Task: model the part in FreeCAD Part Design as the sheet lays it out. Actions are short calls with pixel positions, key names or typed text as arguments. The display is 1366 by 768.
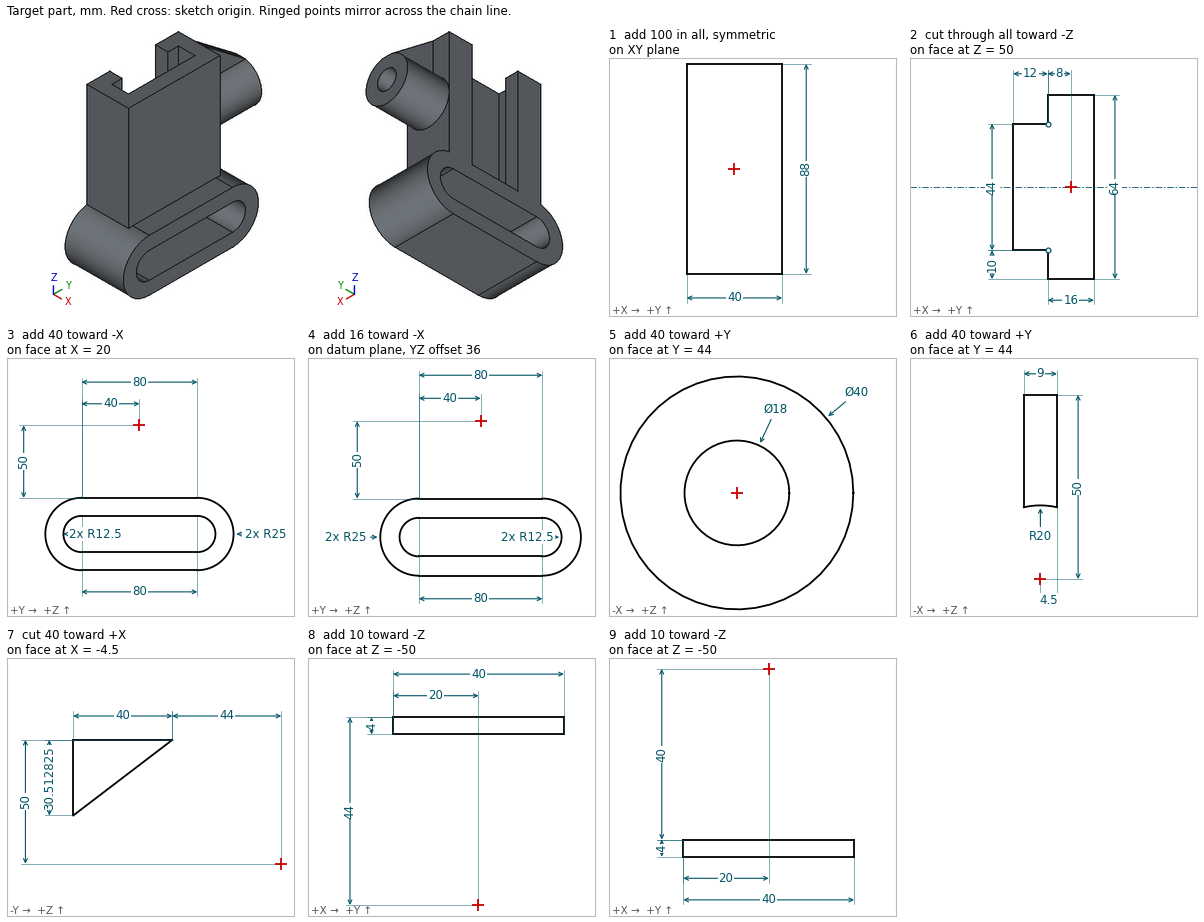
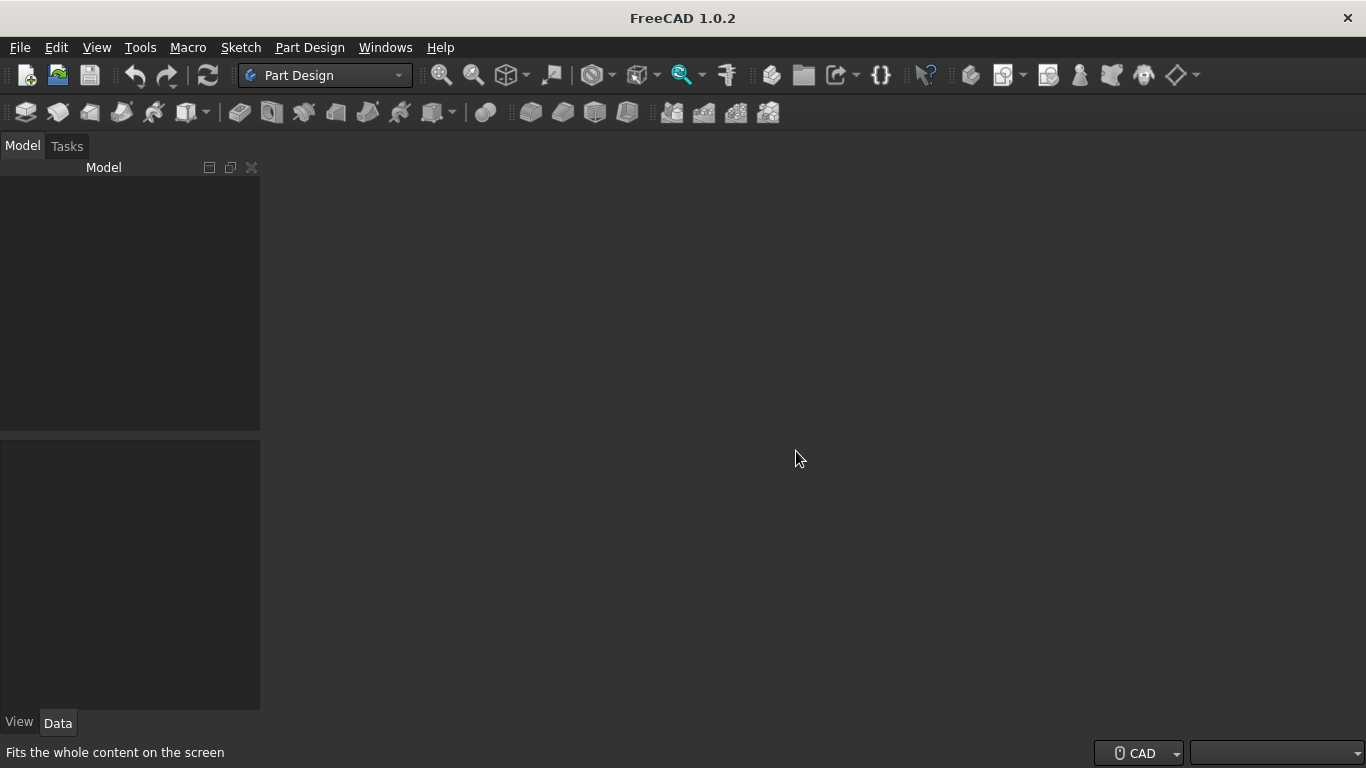
key(ctrl+n)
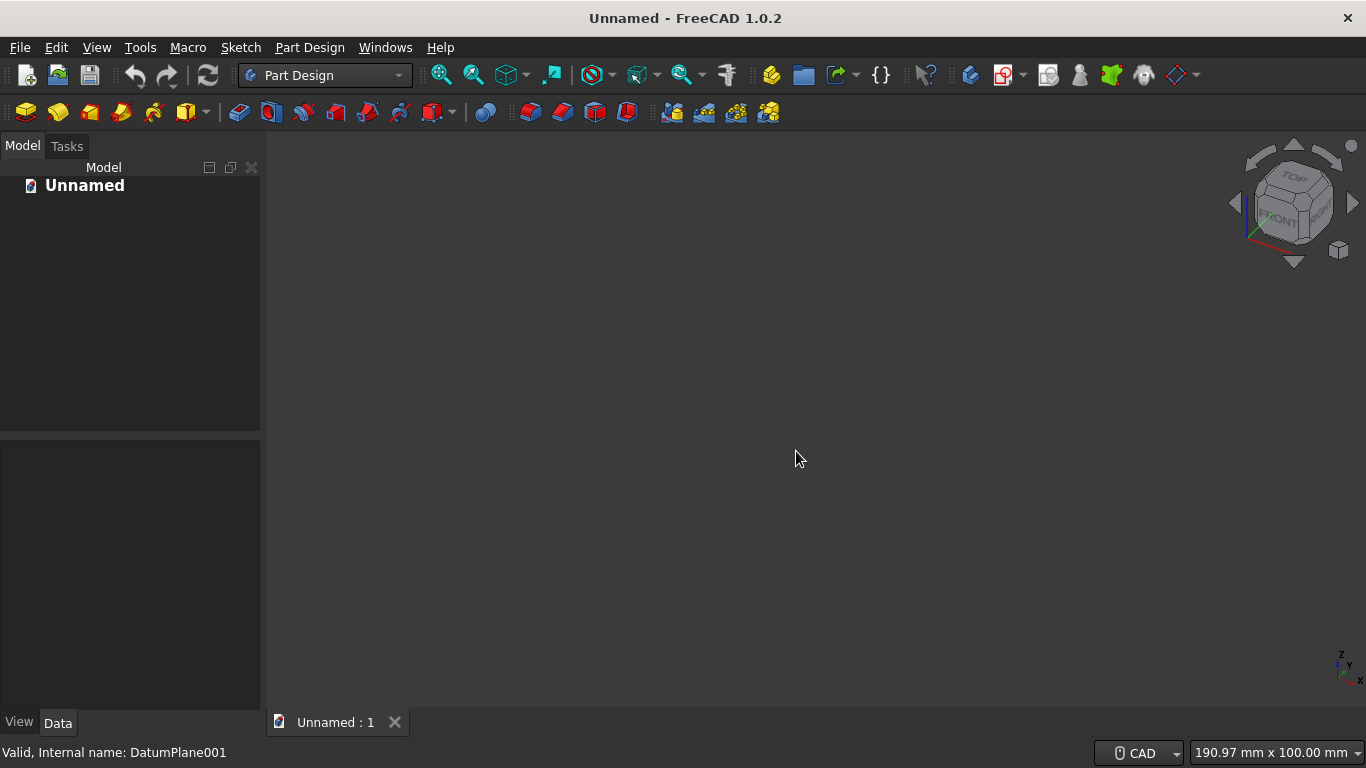
click(1004, 76)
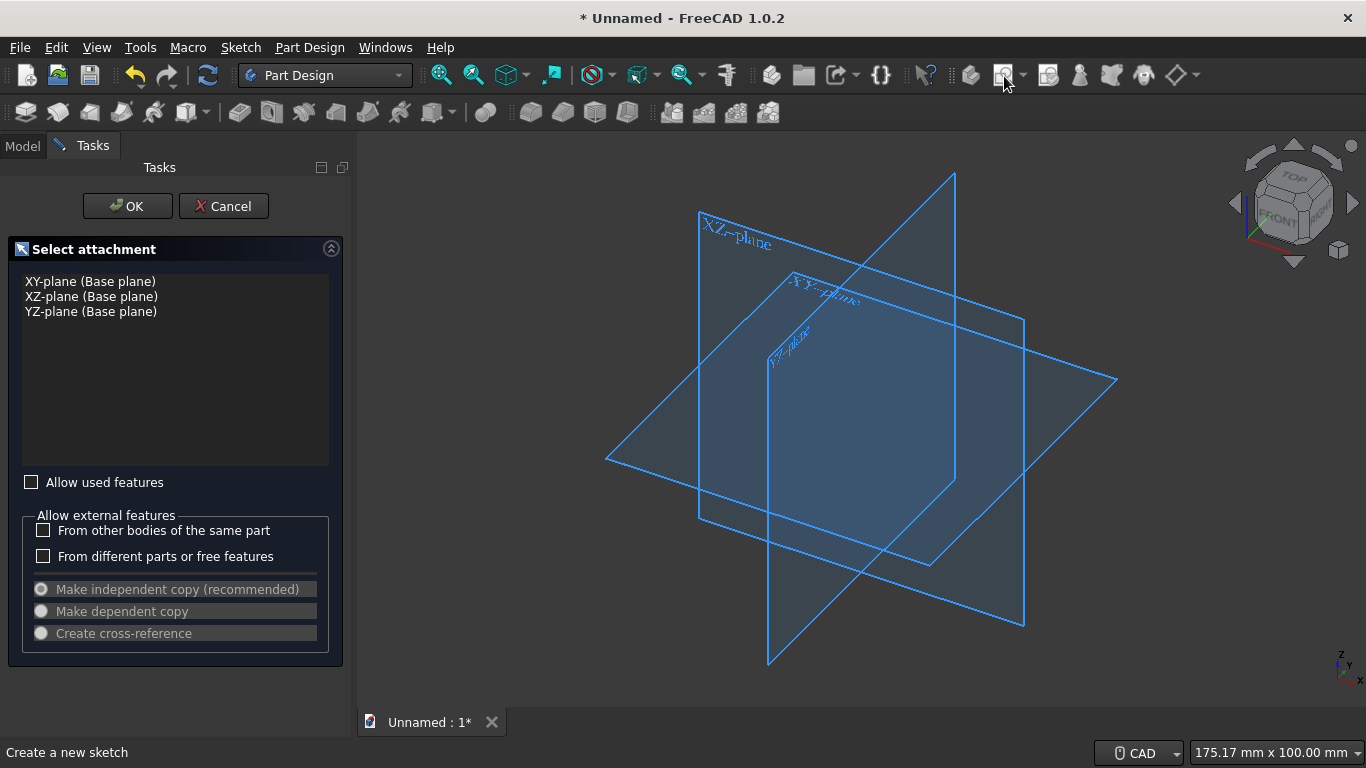
click(82, 282)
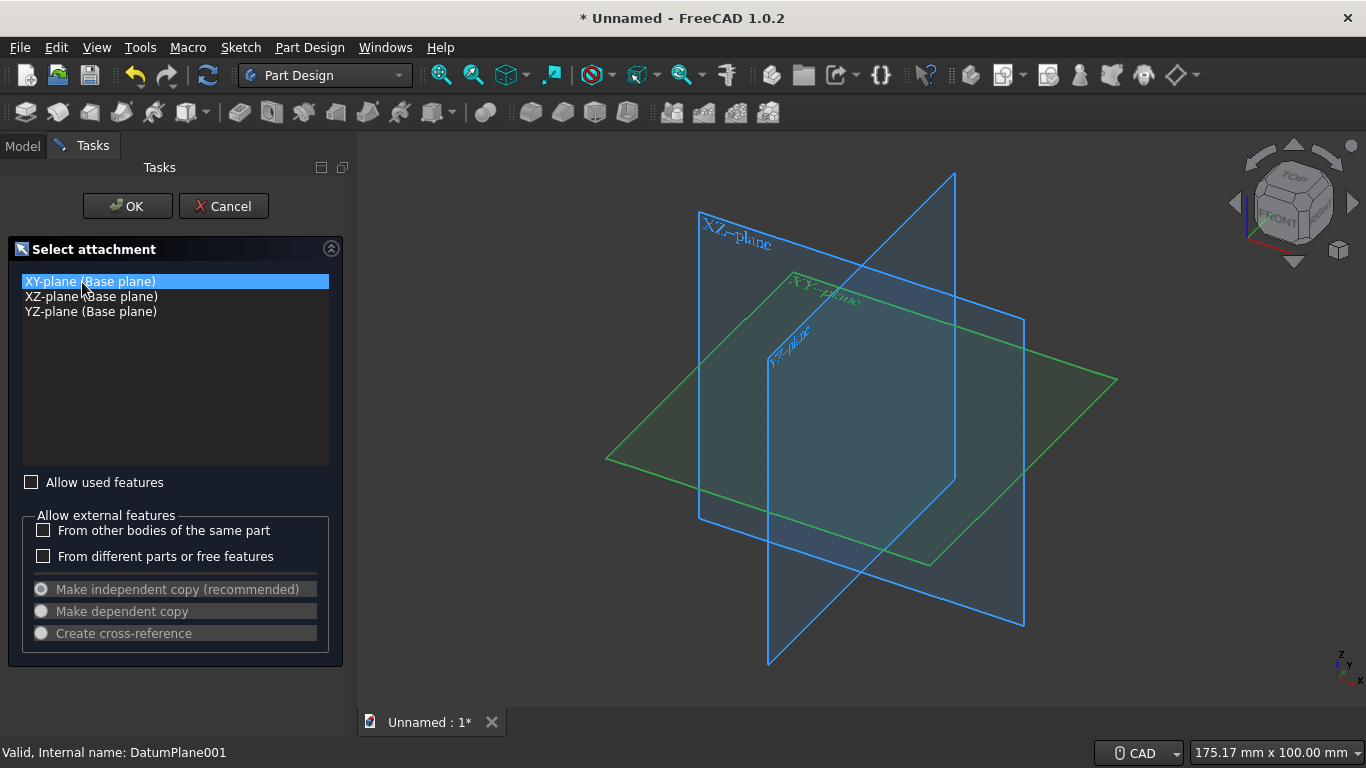
click(128, 206)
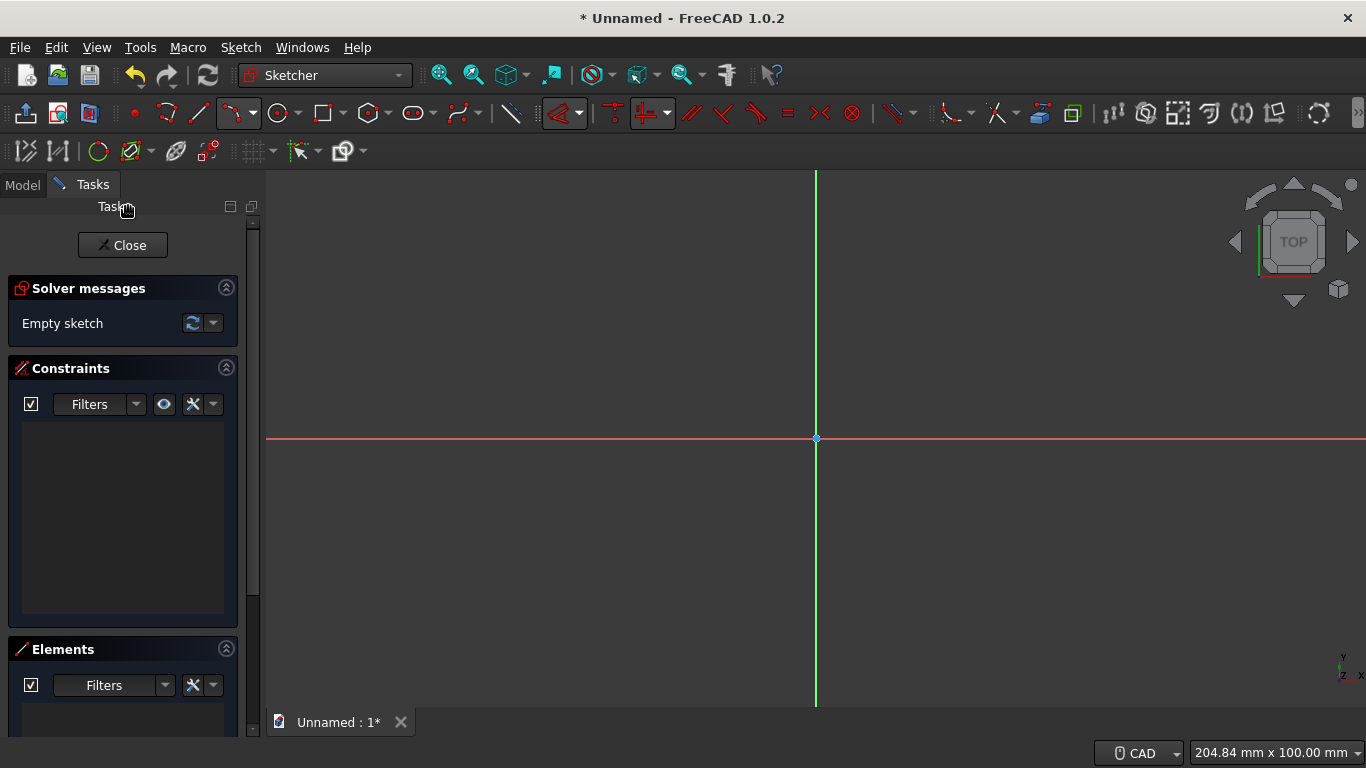
scroll(608, 438, down, 2)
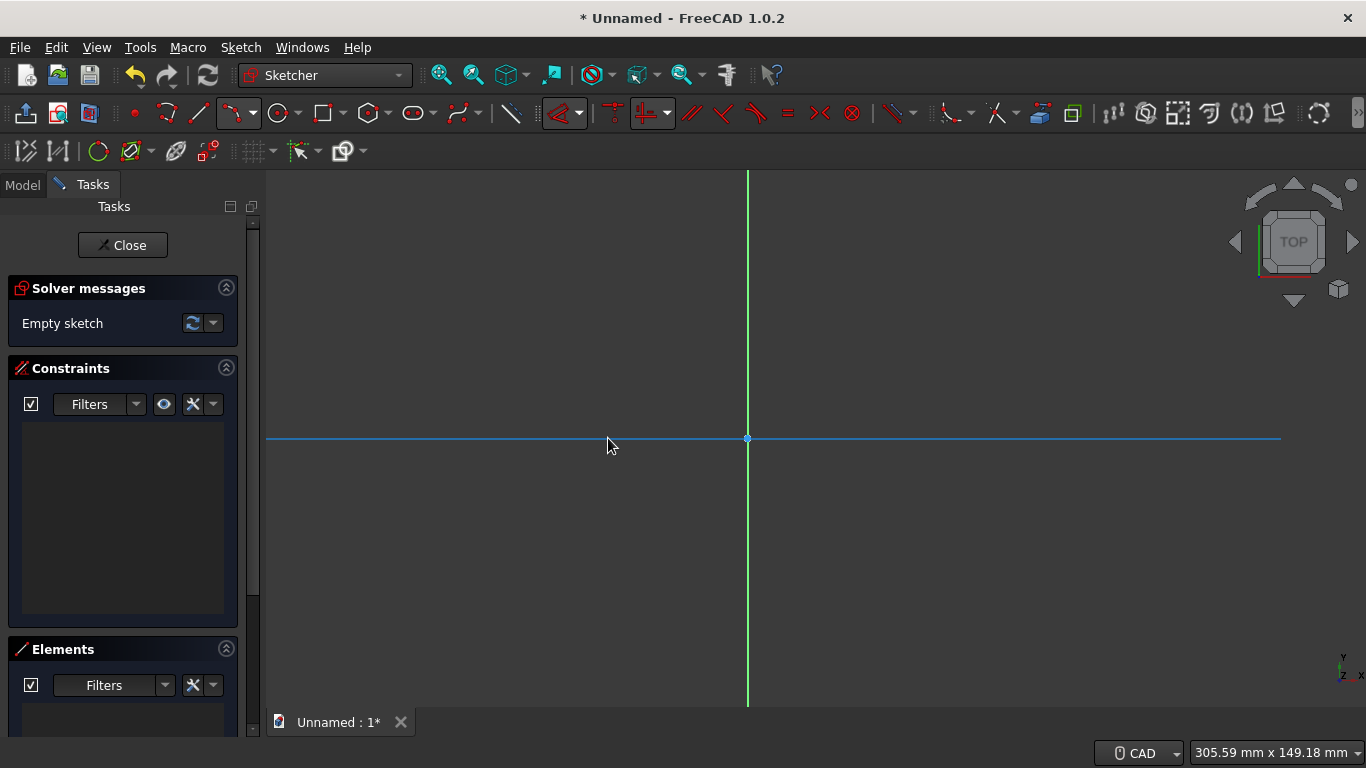
key(g)
key(v)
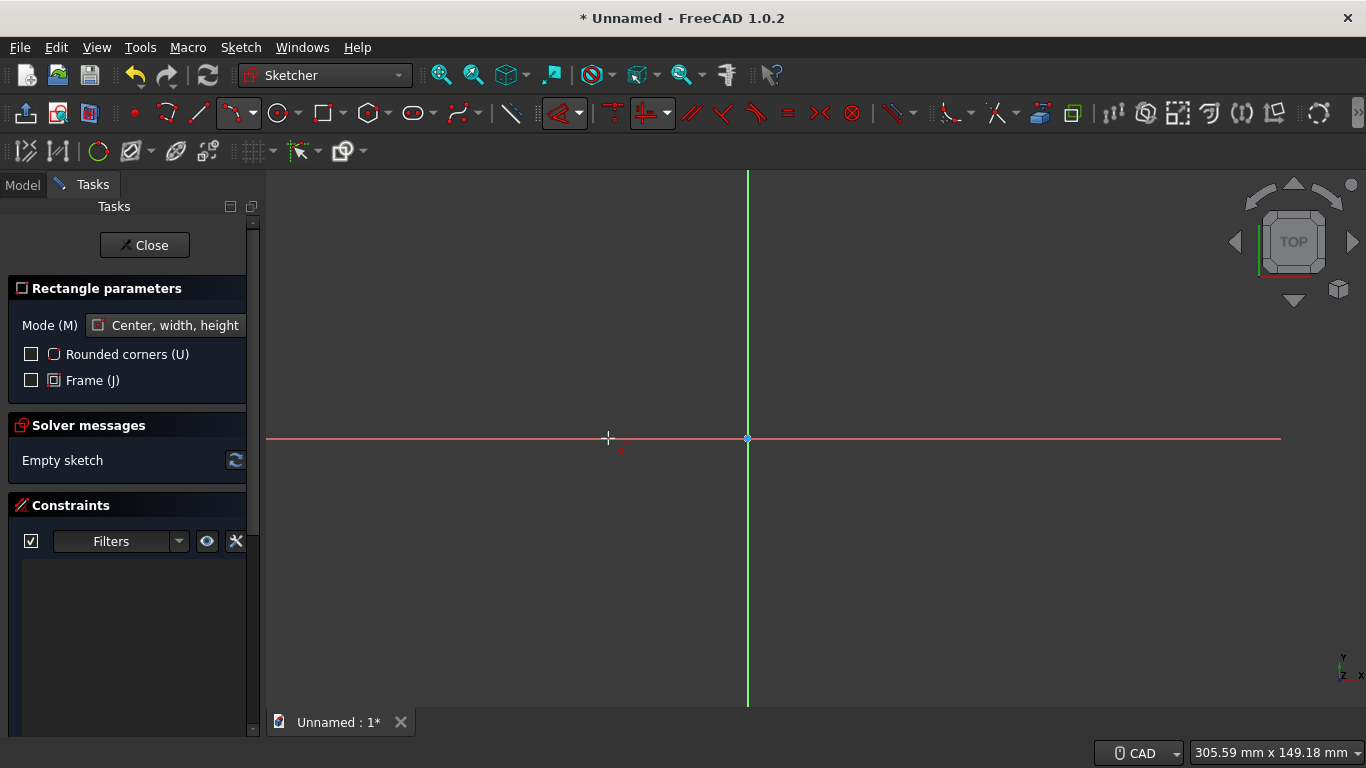
click(748, 438)
click(820, 280)
key(Escape)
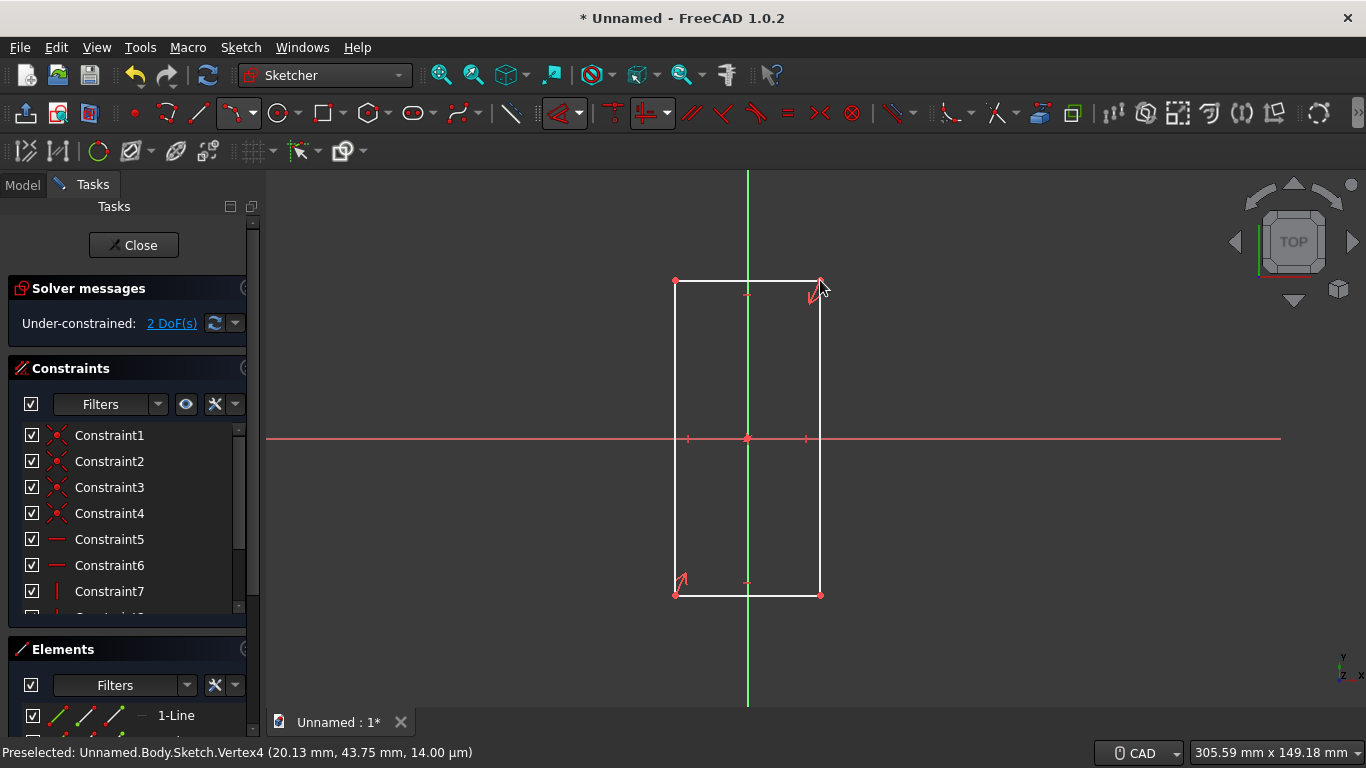
click(719, 596)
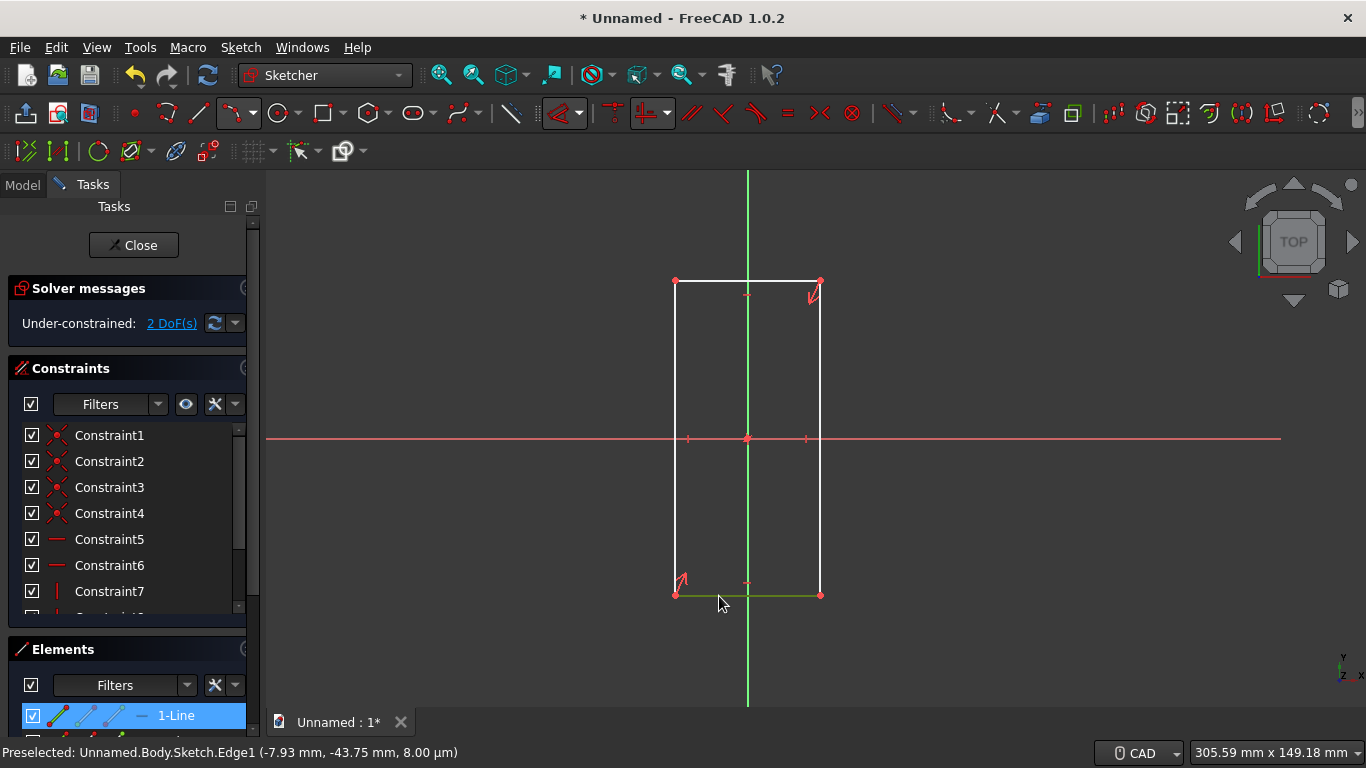
key(l)